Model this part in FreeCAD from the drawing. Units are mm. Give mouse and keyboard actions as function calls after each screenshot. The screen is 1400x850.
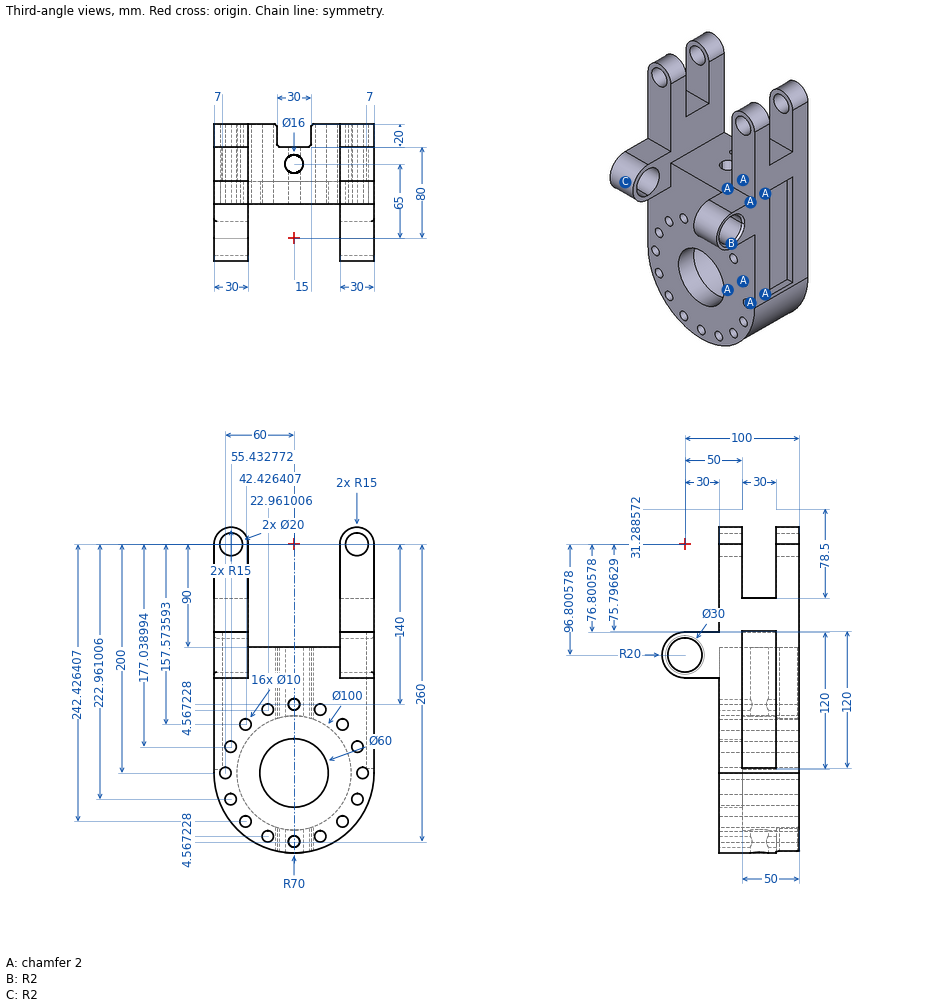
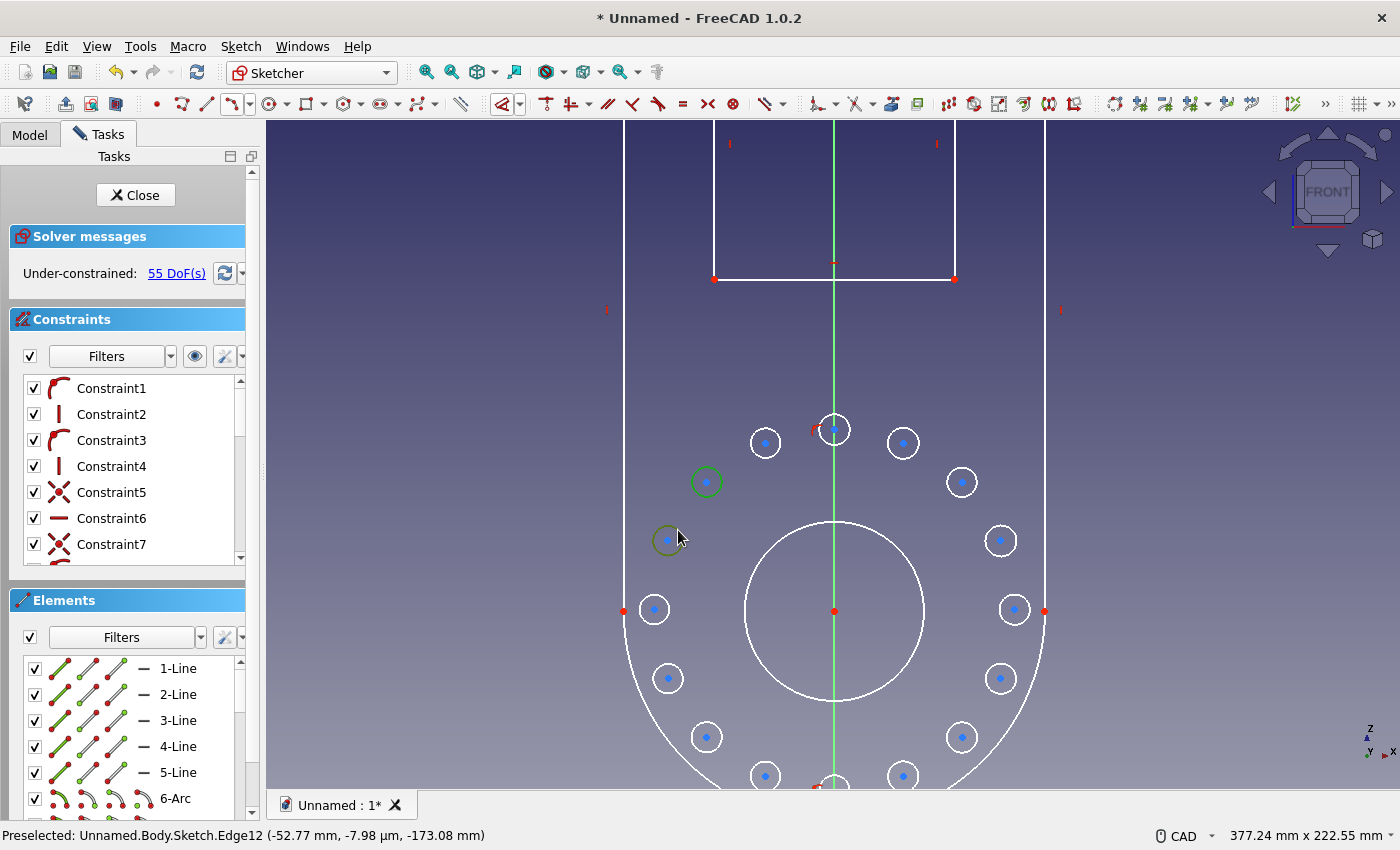
click(776, 433)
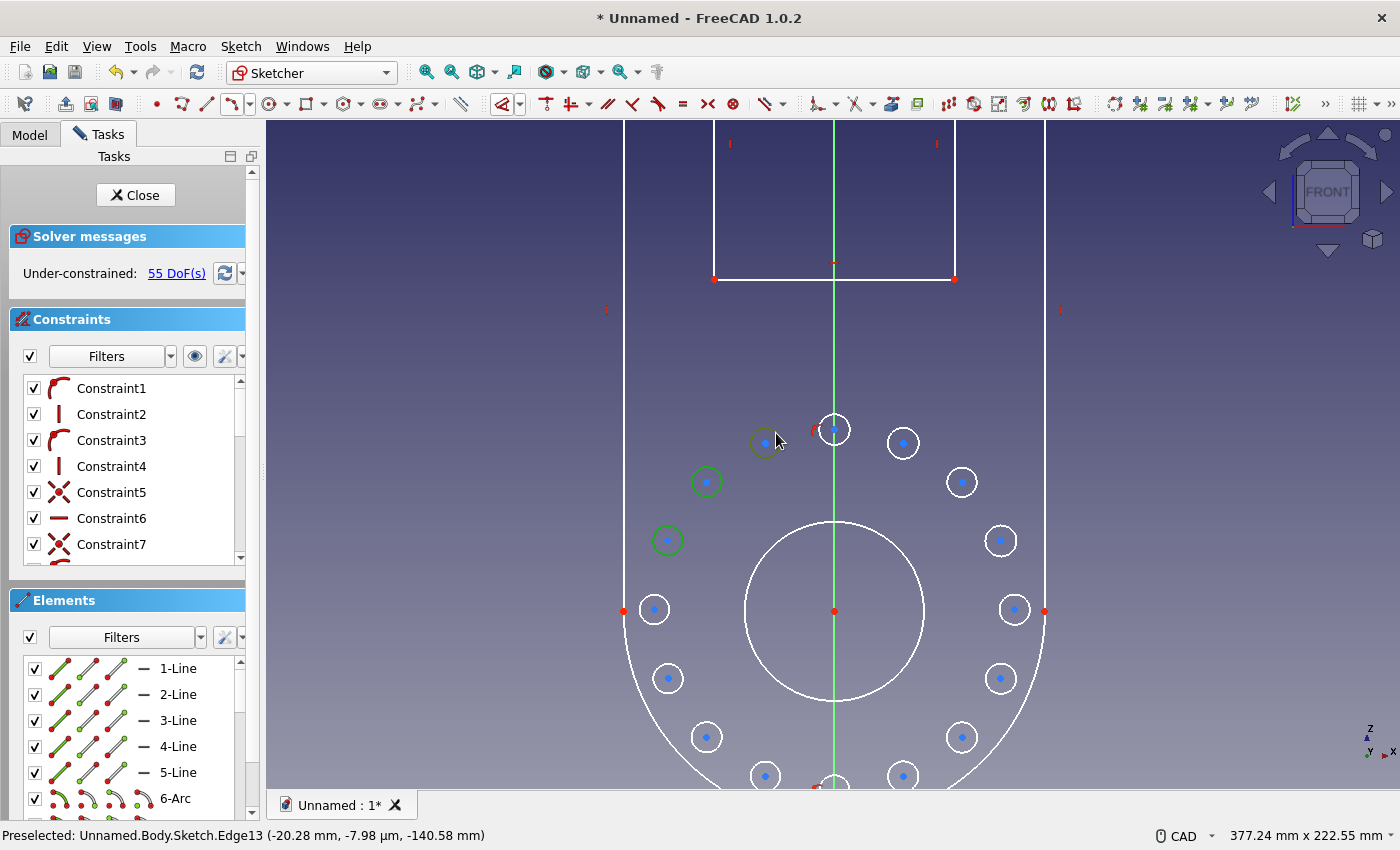
click(665, 599)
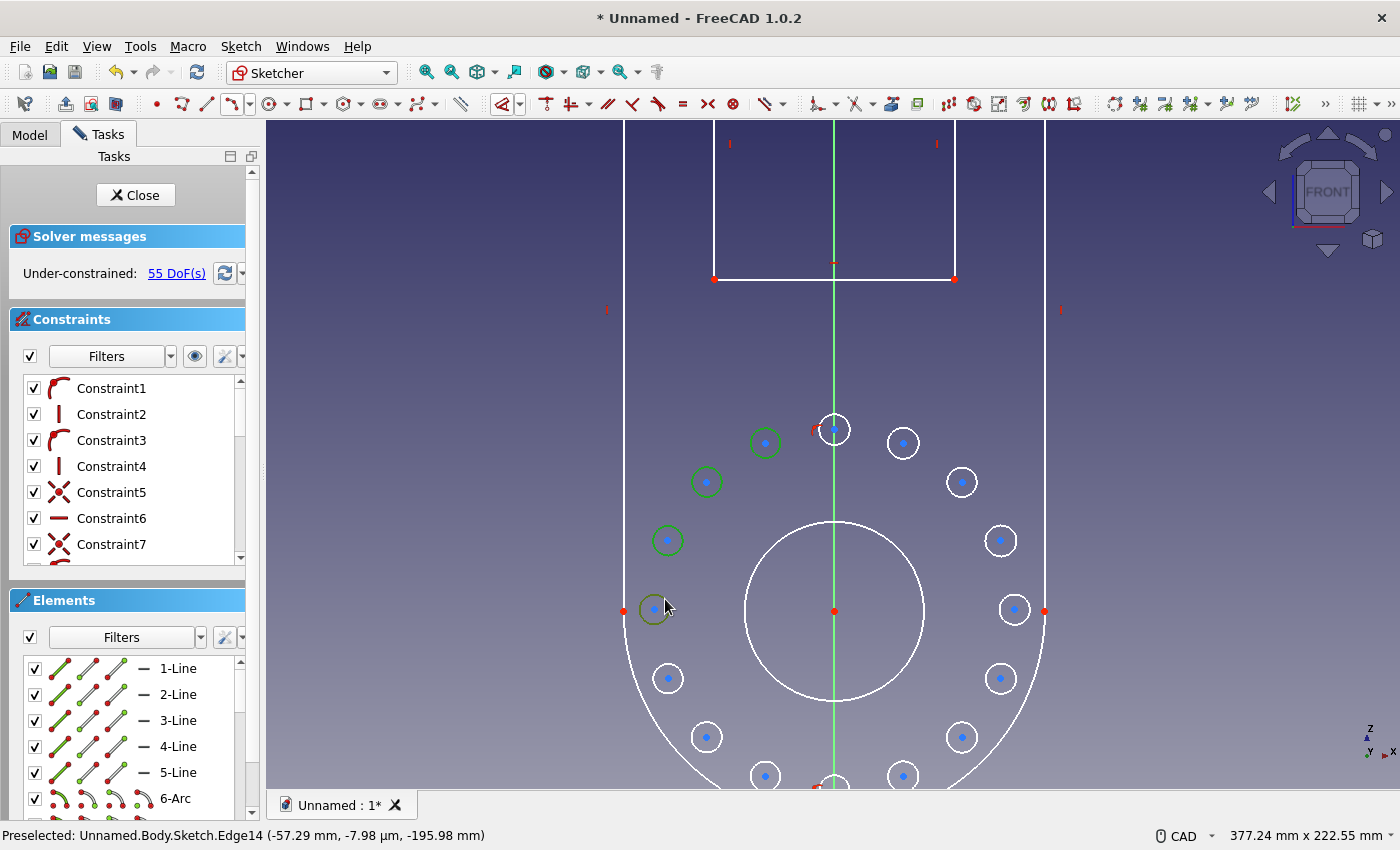
click(678, 668)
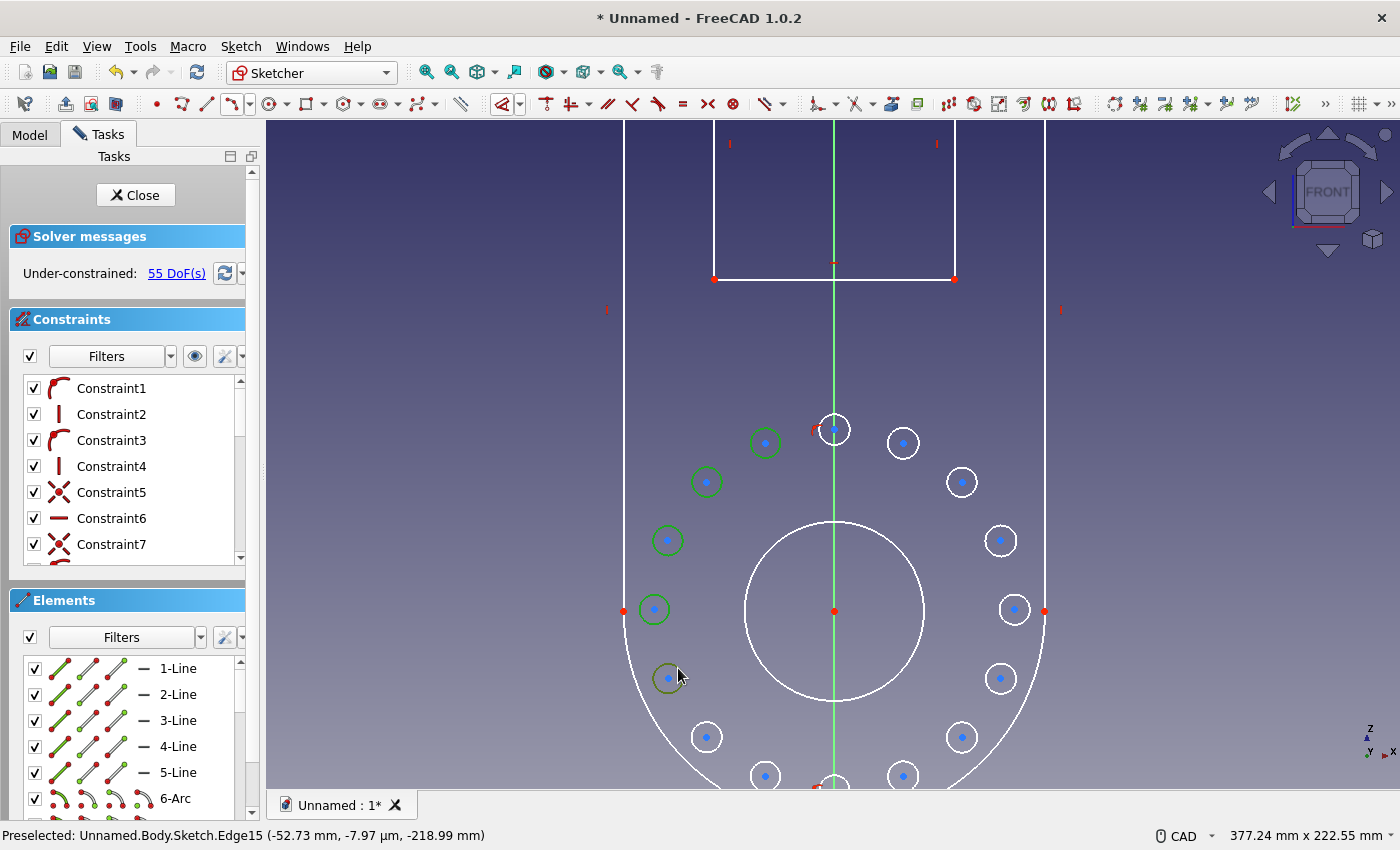
click(717, 727)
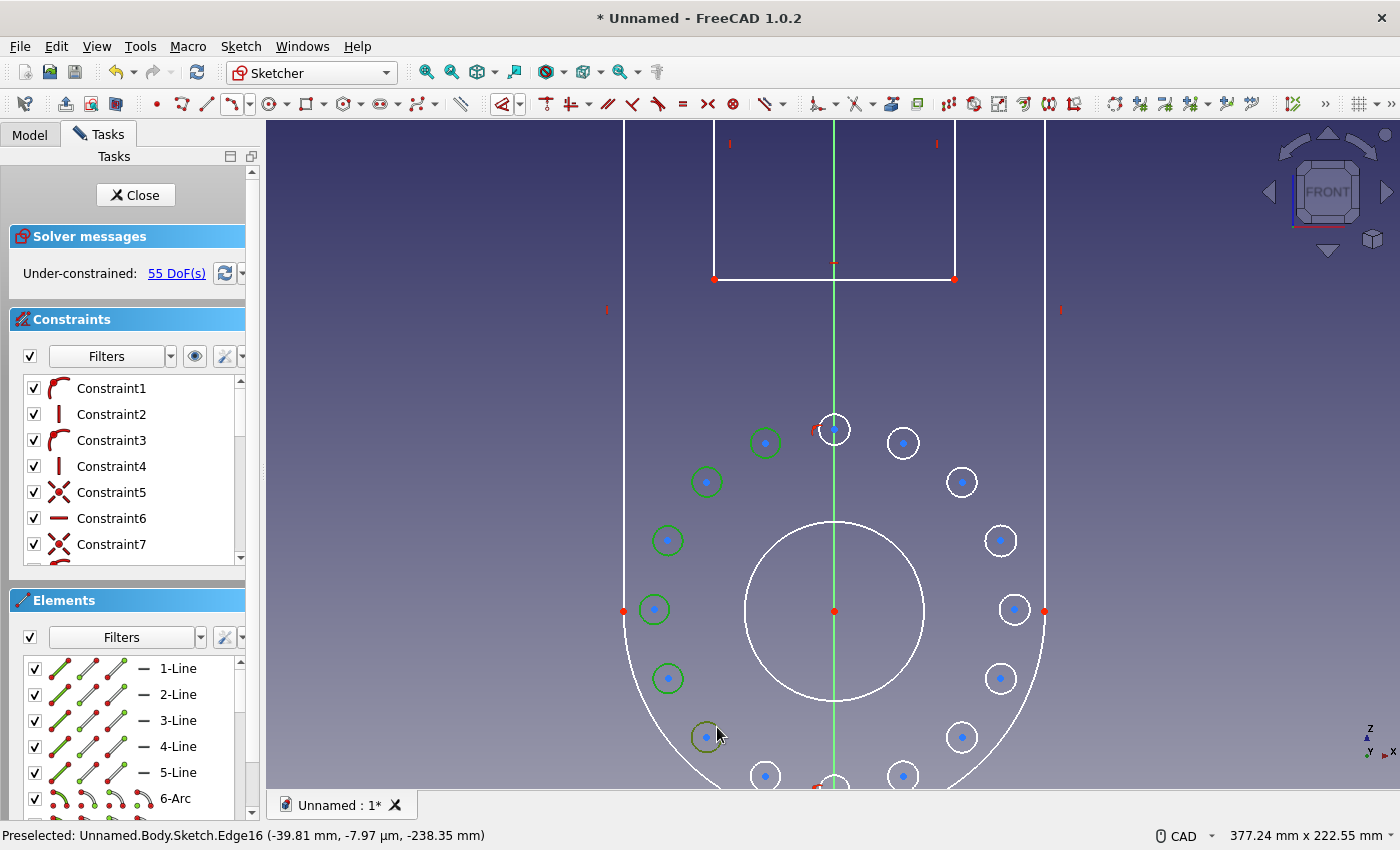
scroll(679, 531, down, 3)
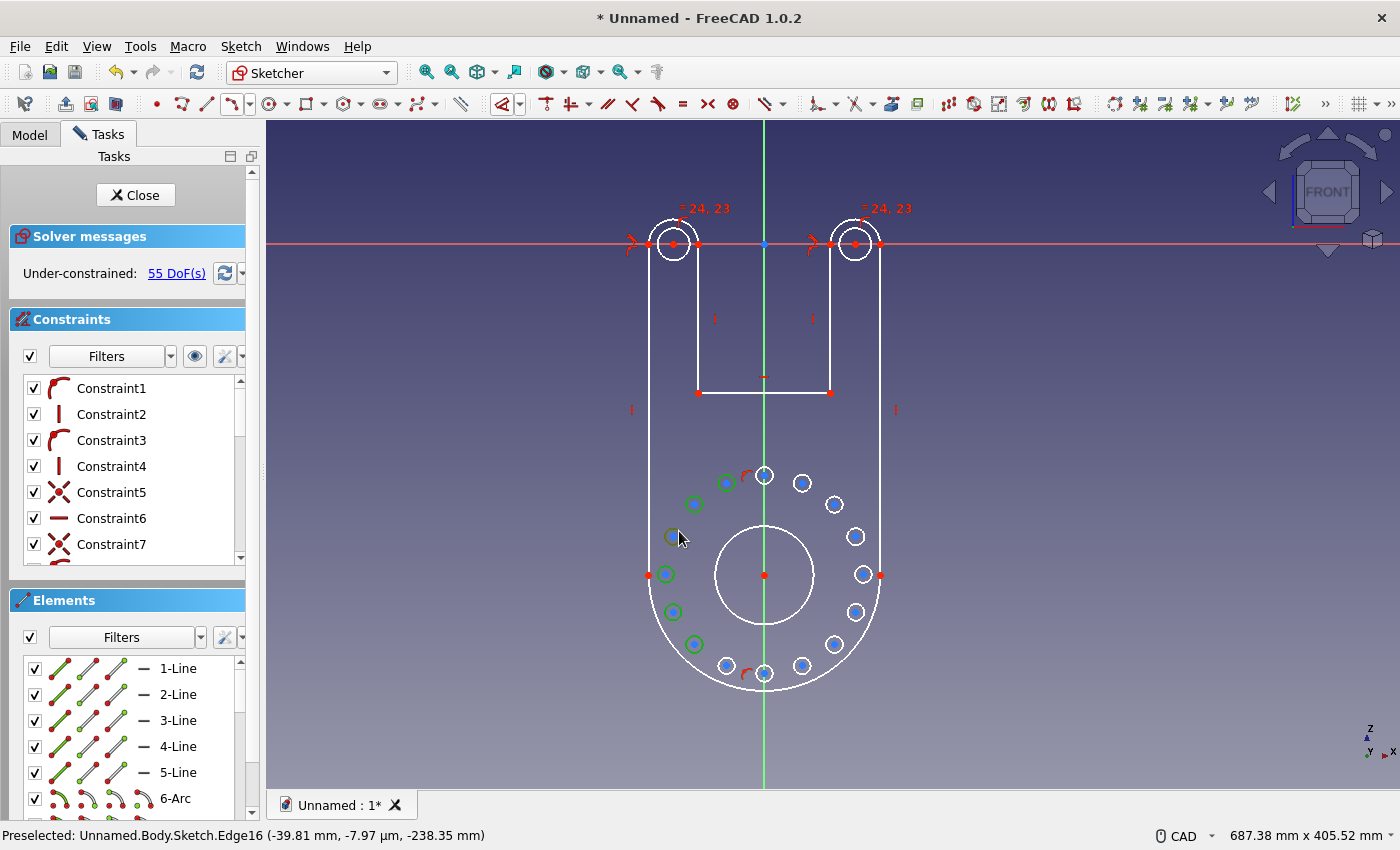
scroll(732, 660, up, 3)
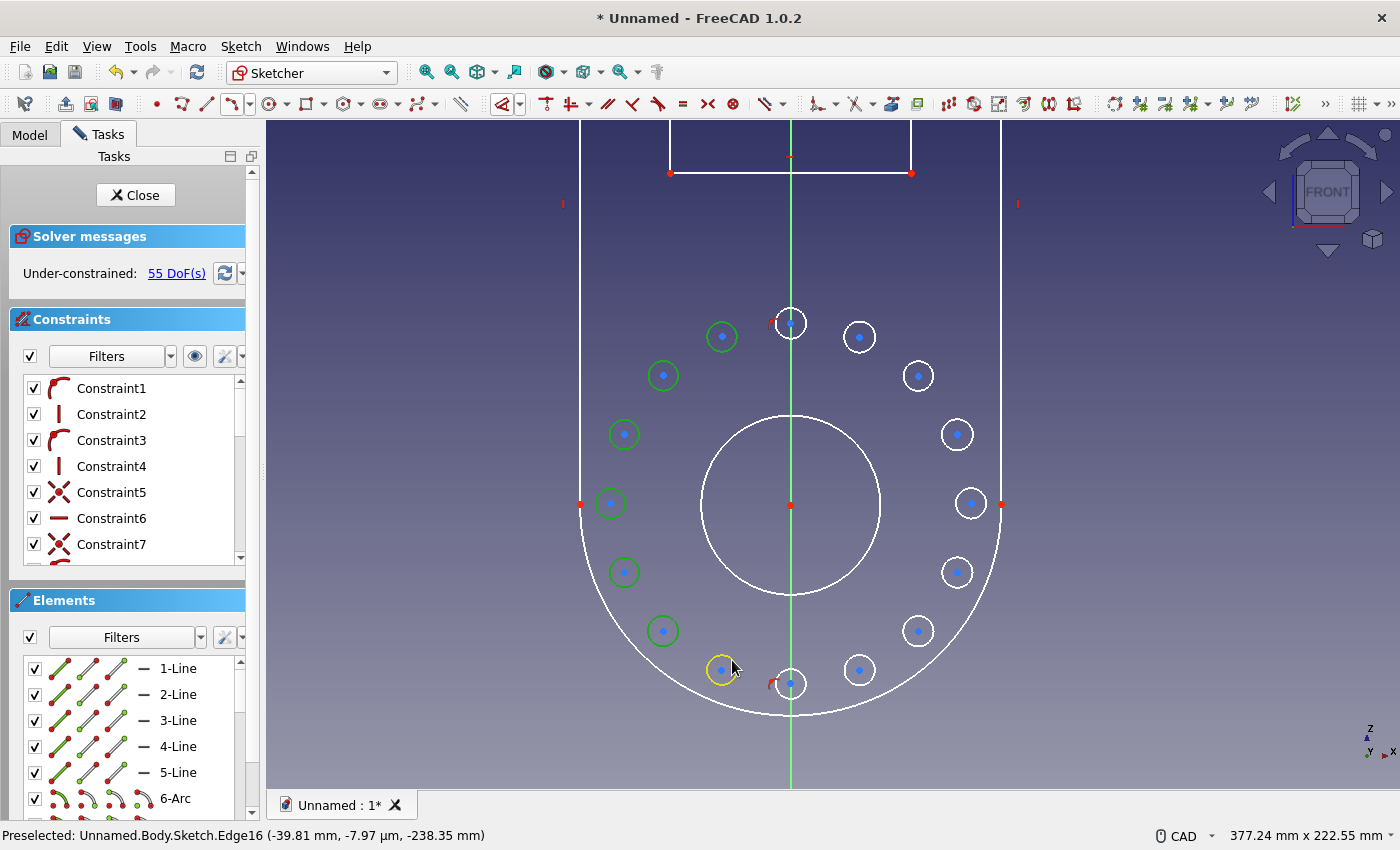
click(732, 660)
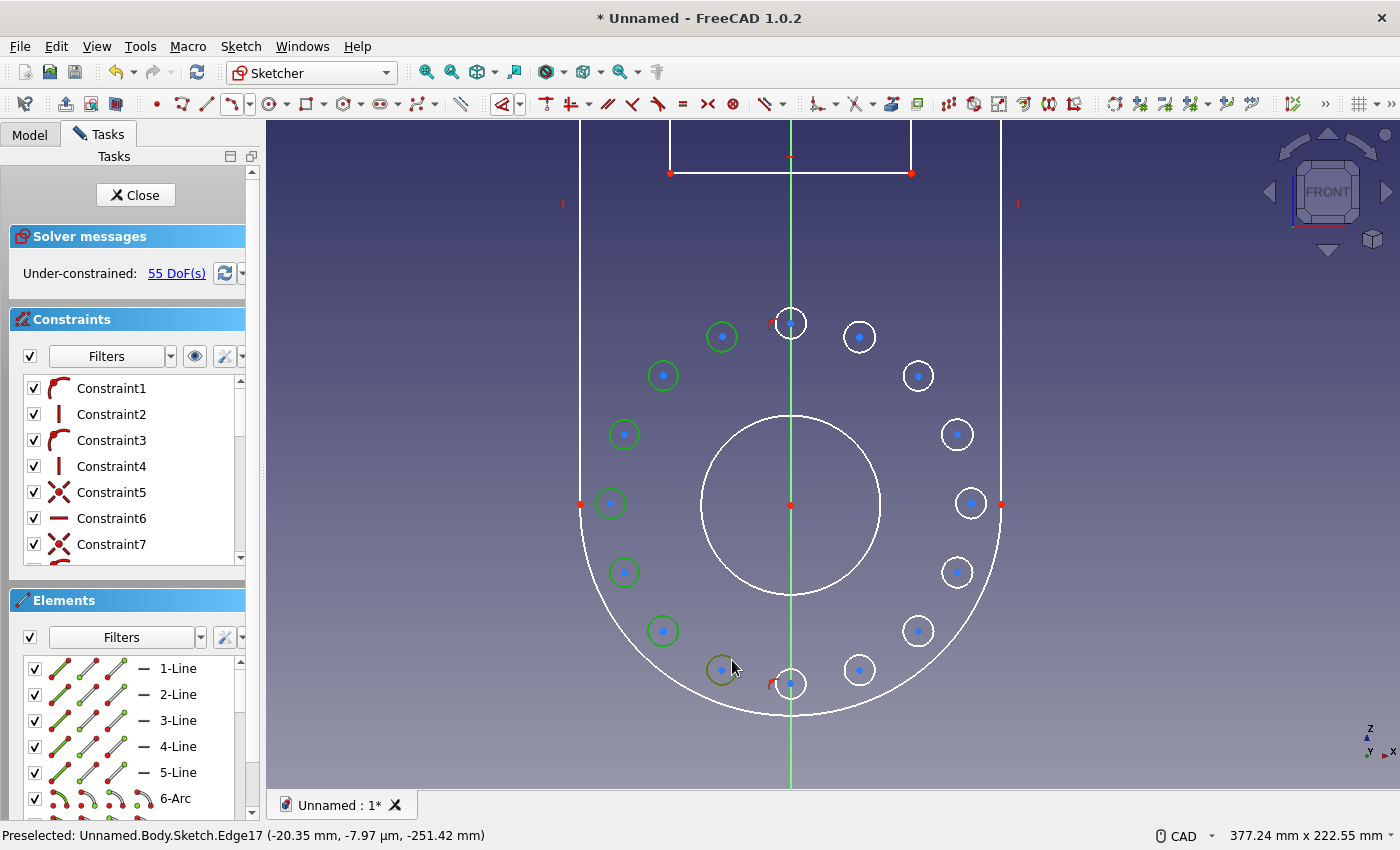
scroll(802, 313, up, 2)